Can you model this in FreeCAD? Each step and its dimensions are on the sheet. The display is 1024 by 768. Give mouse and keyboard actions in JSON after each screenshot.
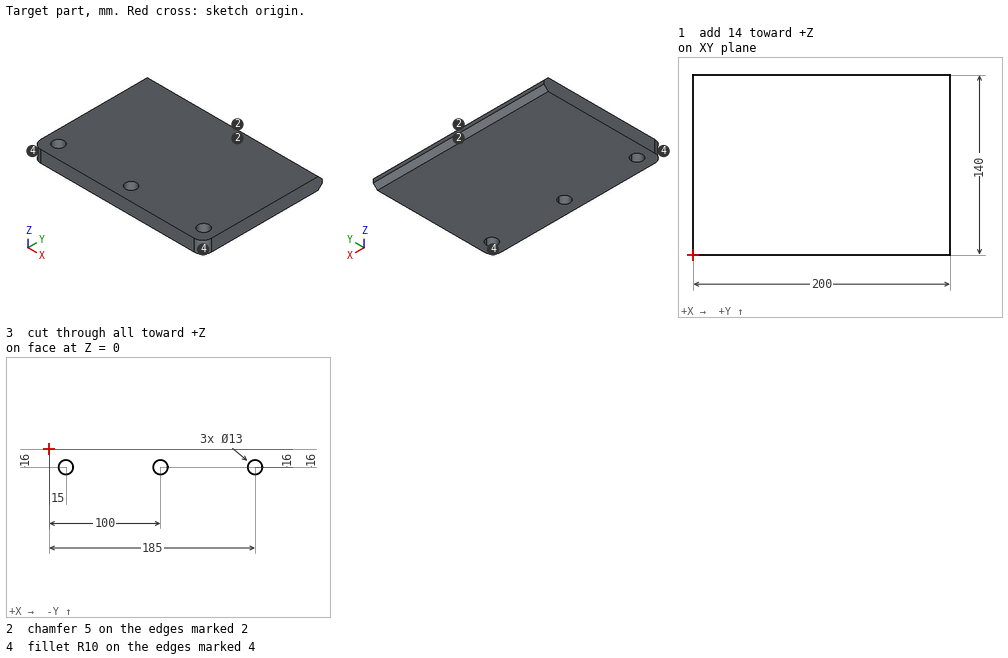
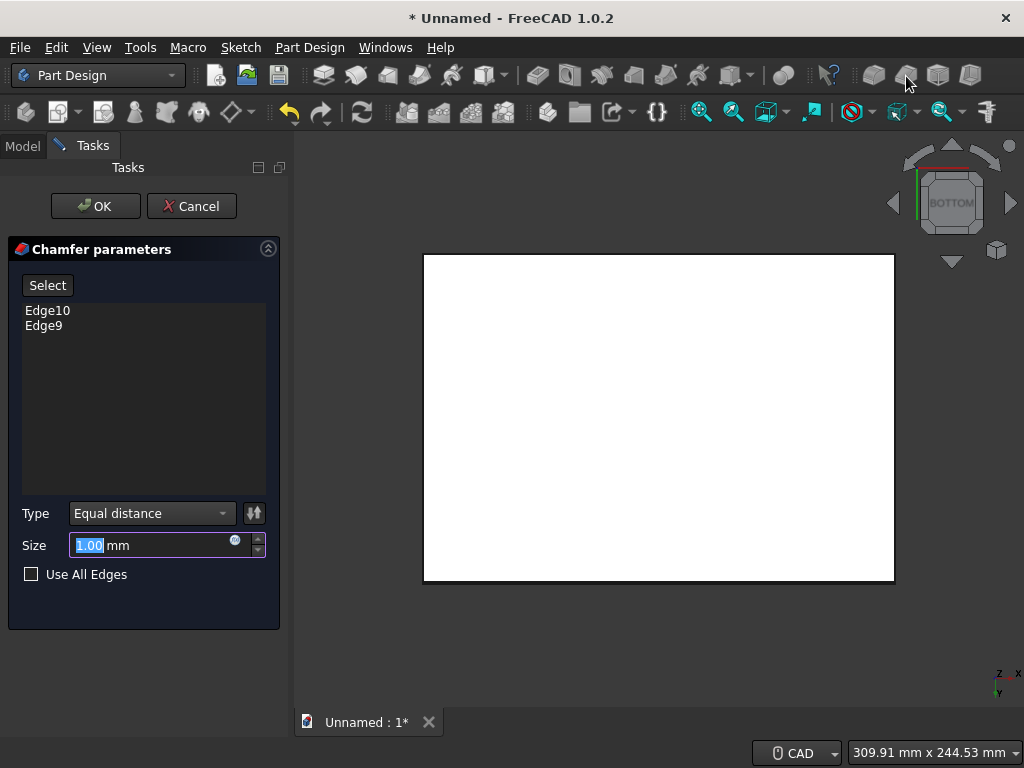
{"action": "type", "text": "5"}
{"action": "key", "text": "Tab"}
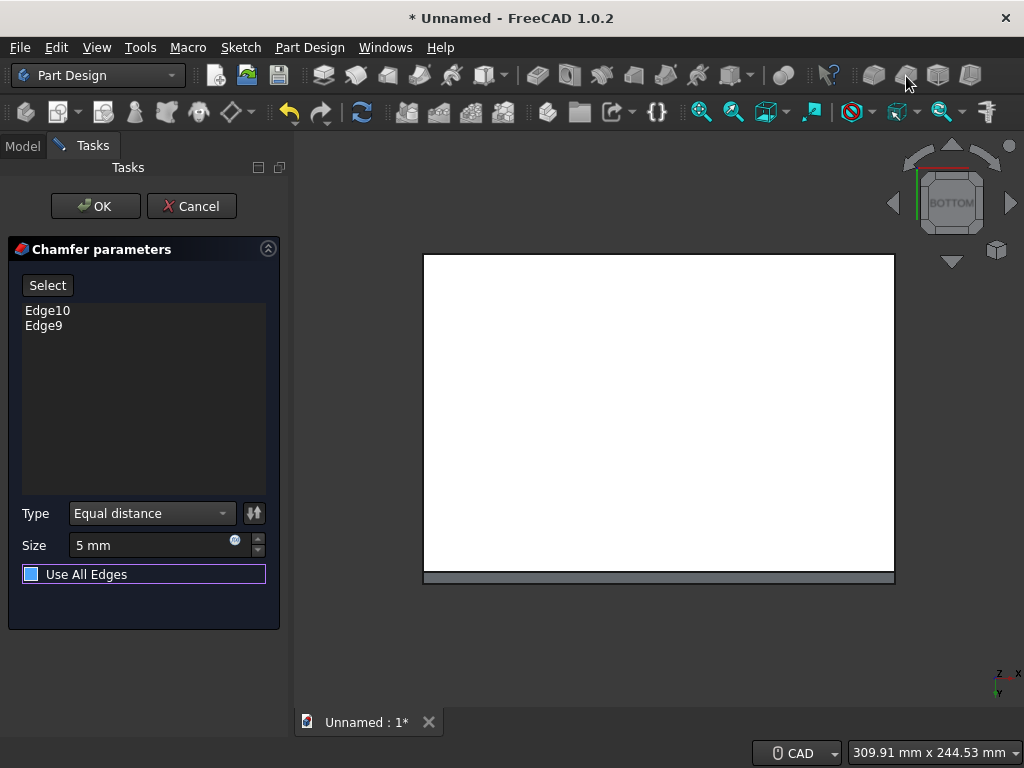
{"action": "left_click", "coordinate": [96, 206]}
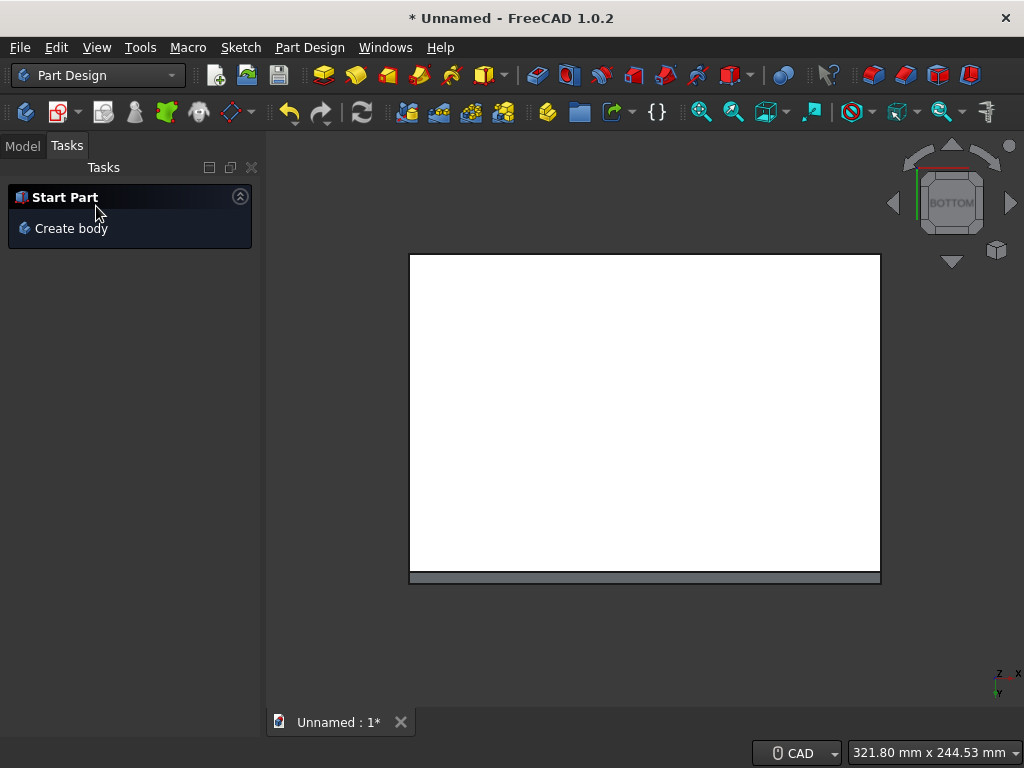
{"action": "left_click", "coordinate": [712, 412]}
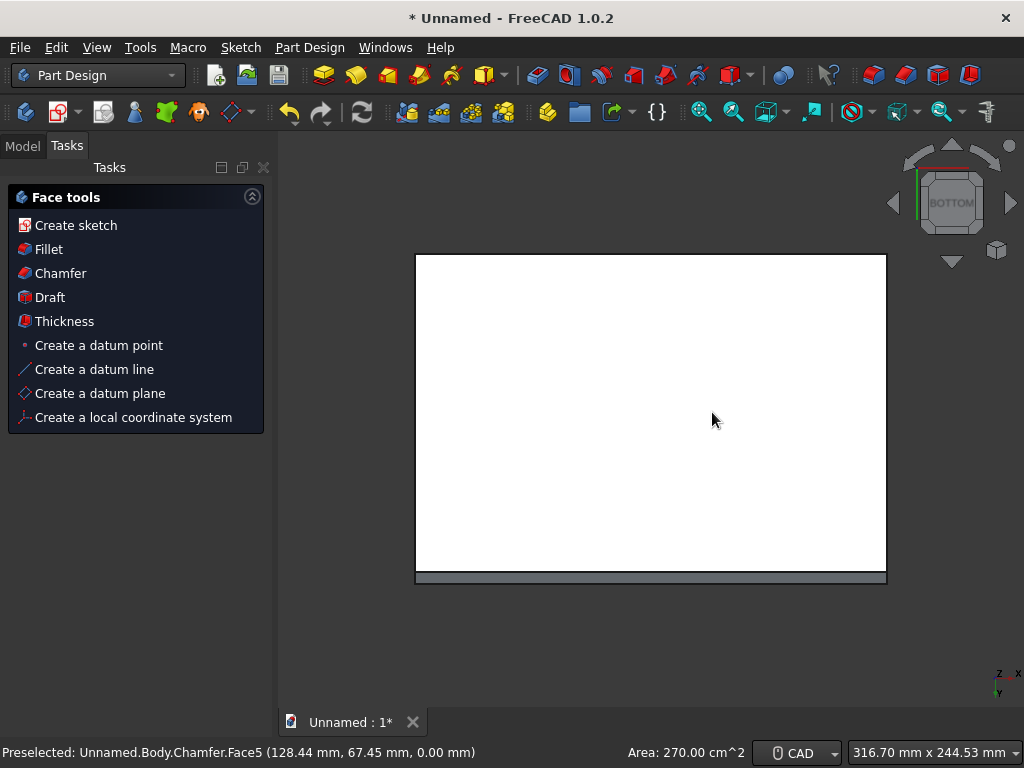
{"action": "left_click", "coordinate": [58, 112]}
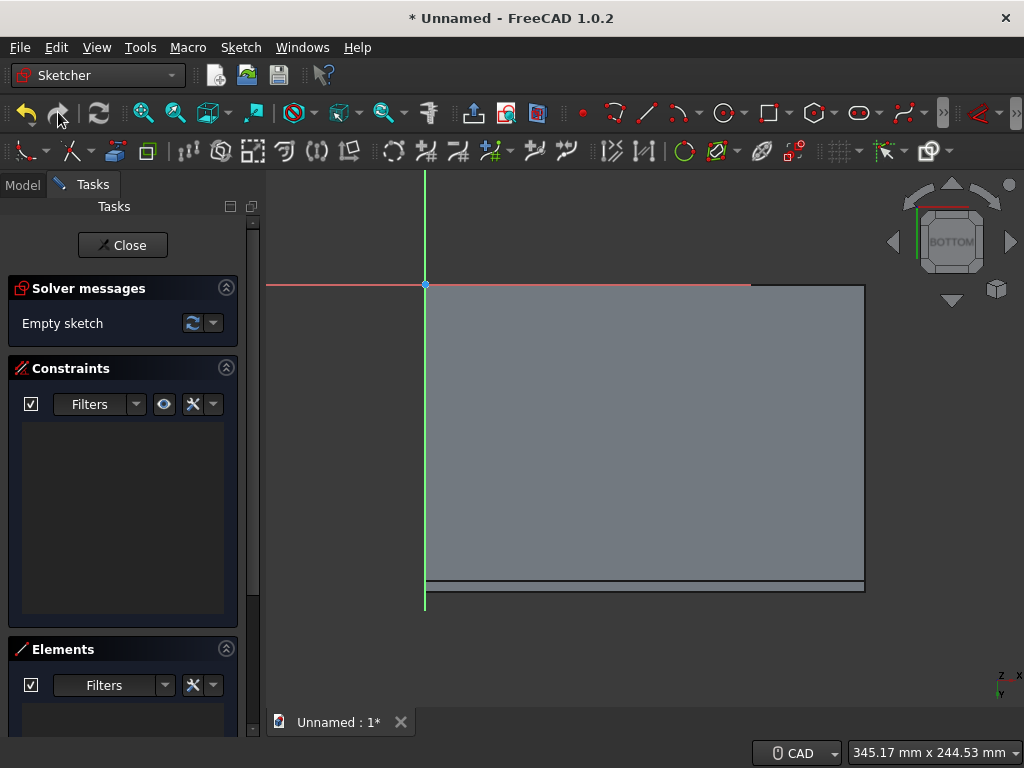
{"action": "scroll", "coordinate": [309, 679], "scroll_direction": "down", "scroll_amount": 1}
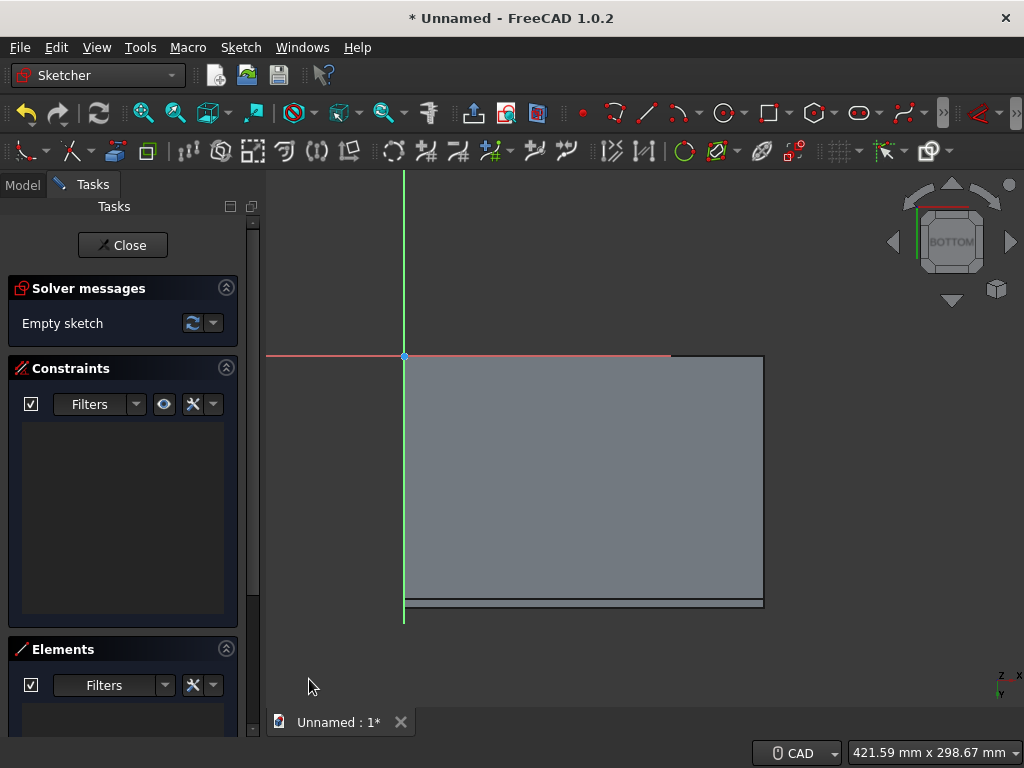
{"action": "left_click", "coordinate": [724, 114]}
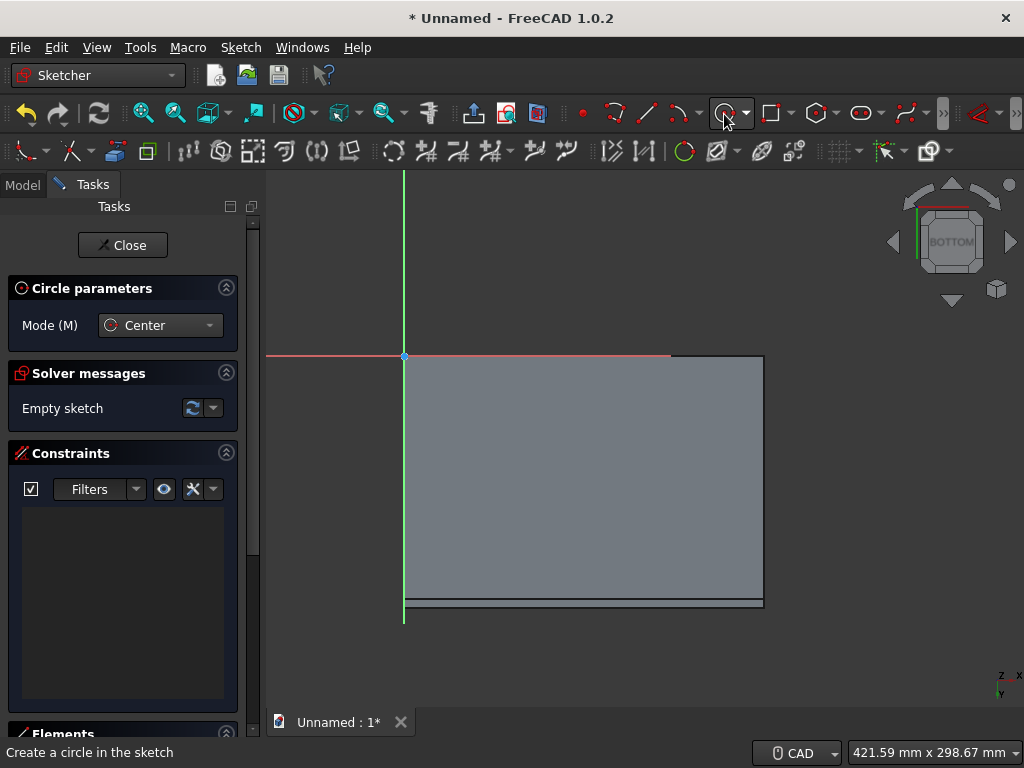
{"action": "scroll", "coordinate": [737, 385], "scroll_direction": "up", "scroll_amount": 4}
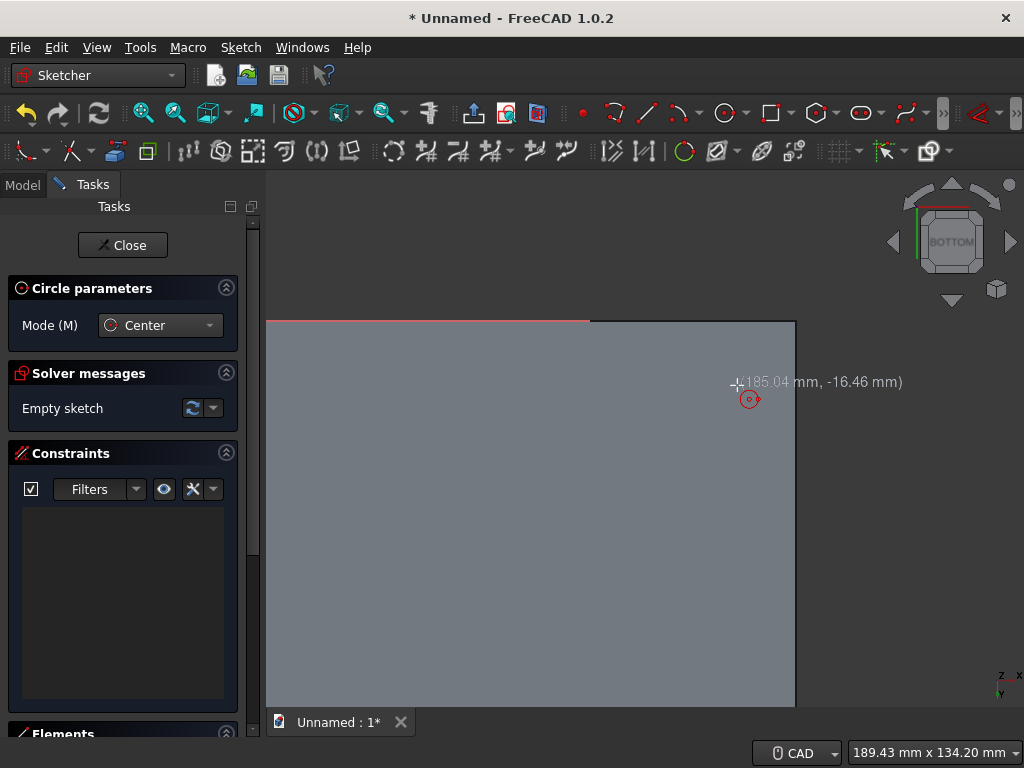
{"action": "left_click", "coordinate": [736, 385]}
{"action": "left_click", "coordinate": [754, 367]}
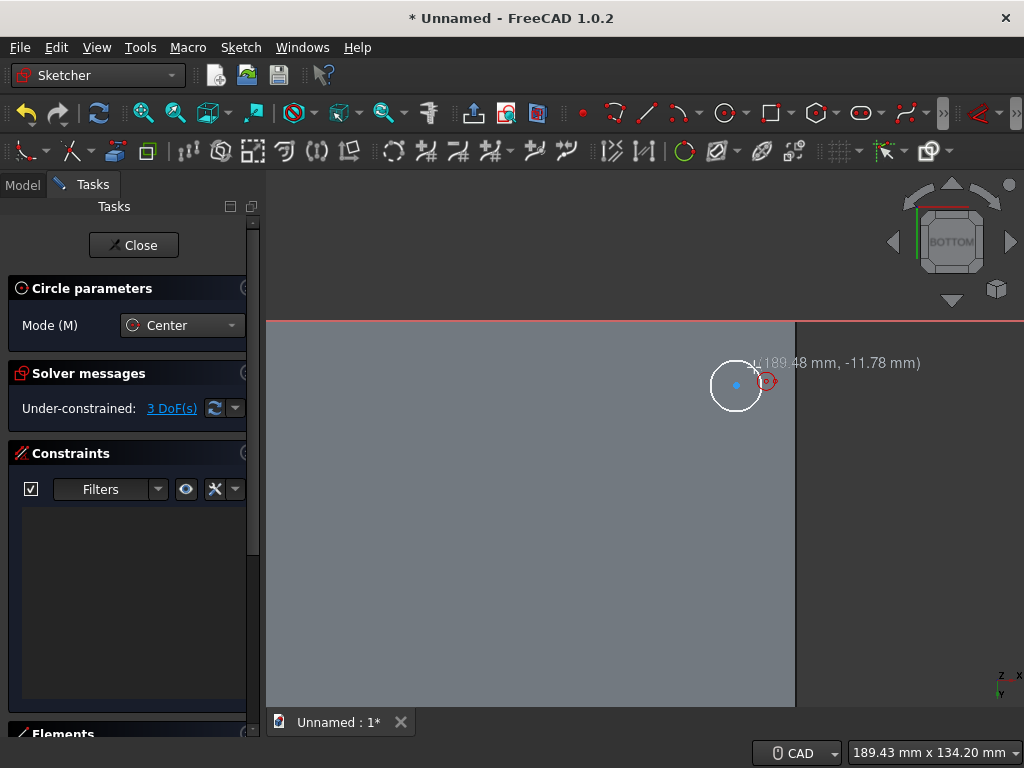
{"action": "left_click", "coordinate": [396, 385]}
{"action": "left_click", "coordinate": [414, 367]}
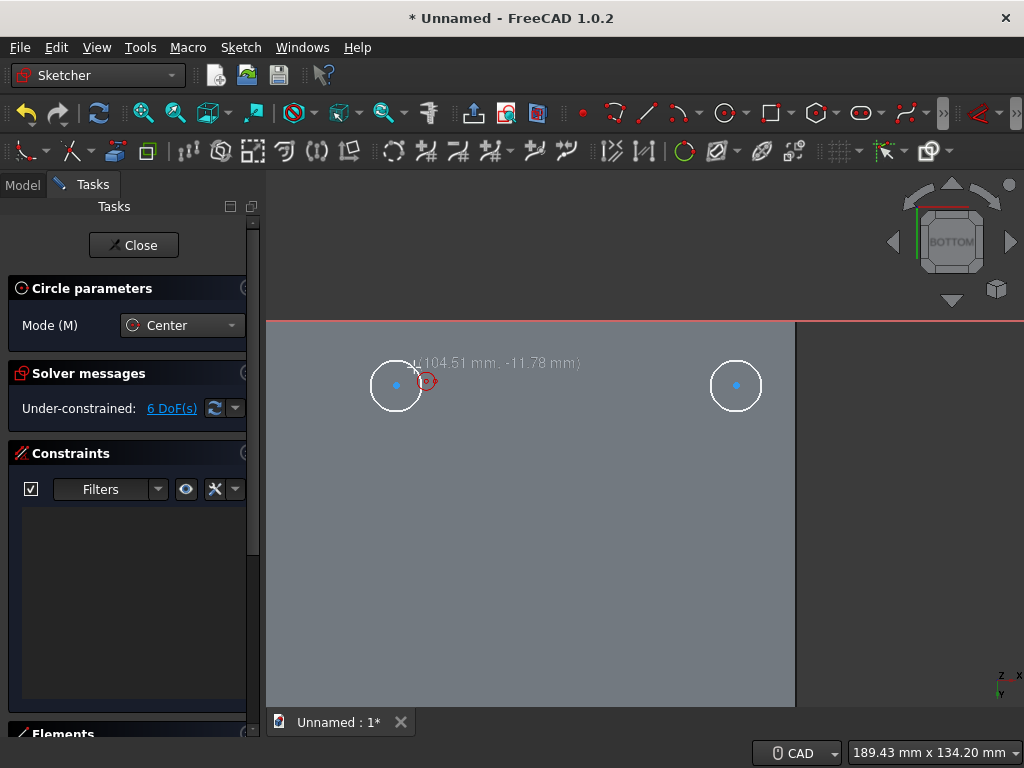
{"action": "scroll", "coordinate": [817, 527], "scroll_direction": "down", "scroll_amount": 3}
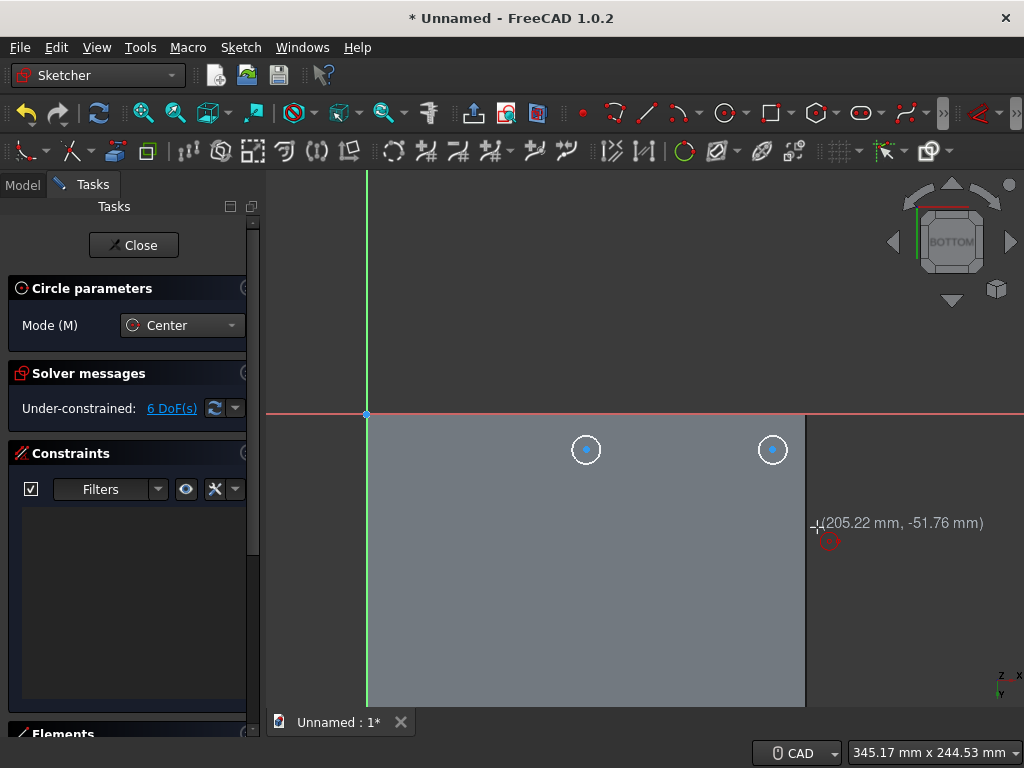
{"action": "scroll", "coordinate": [400, 449], "scroll_direction": "up", "scroll_amount": 3}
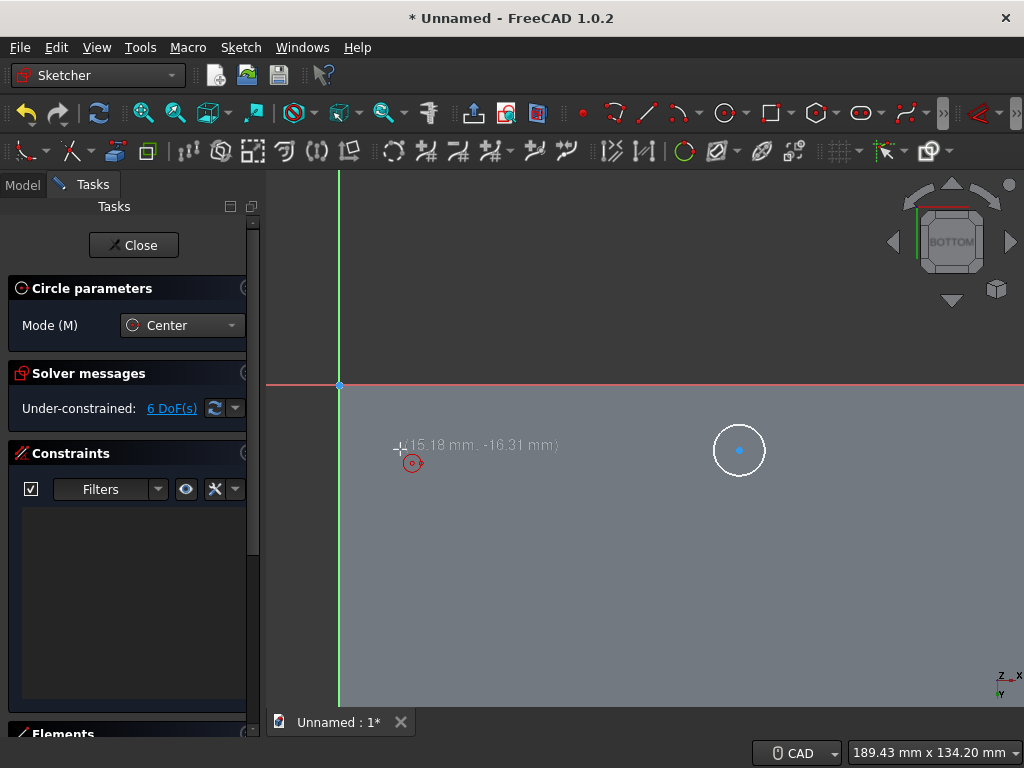
{"action": "left_click", "coordinate": [399, 449]}
{"action": "left_click", "coordinate": [418, 431]}
{"action": "key", "text": "Escape"}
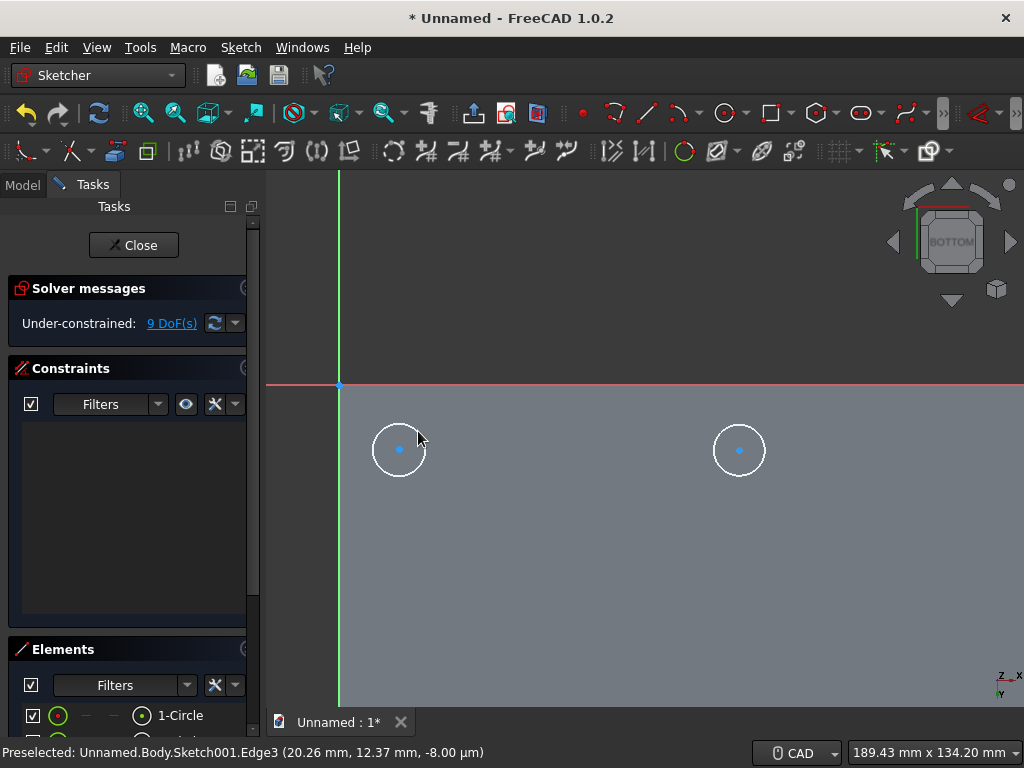
{"action": "scroll", "coordinate": [399, 449], "scroll_direction": "down", "scroll_amount": 3}